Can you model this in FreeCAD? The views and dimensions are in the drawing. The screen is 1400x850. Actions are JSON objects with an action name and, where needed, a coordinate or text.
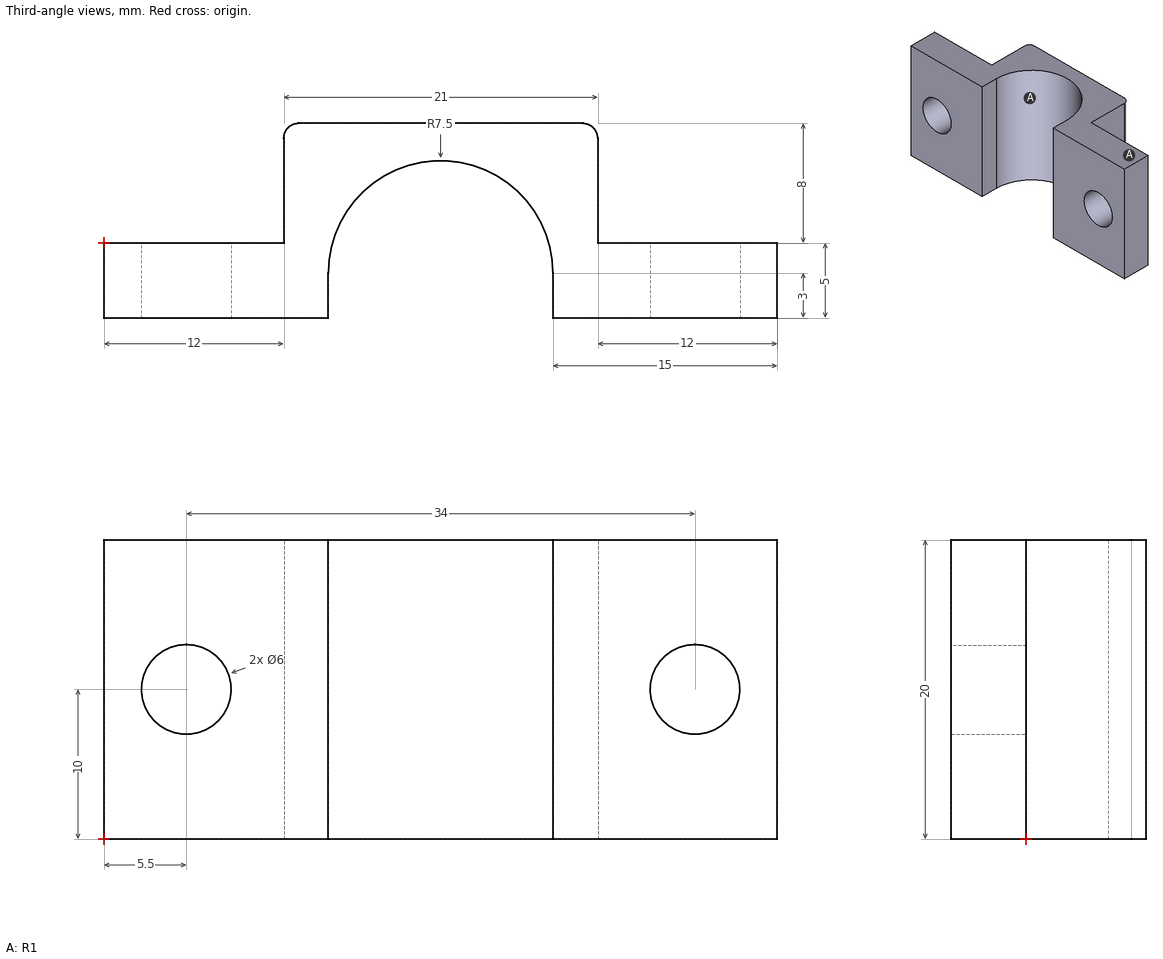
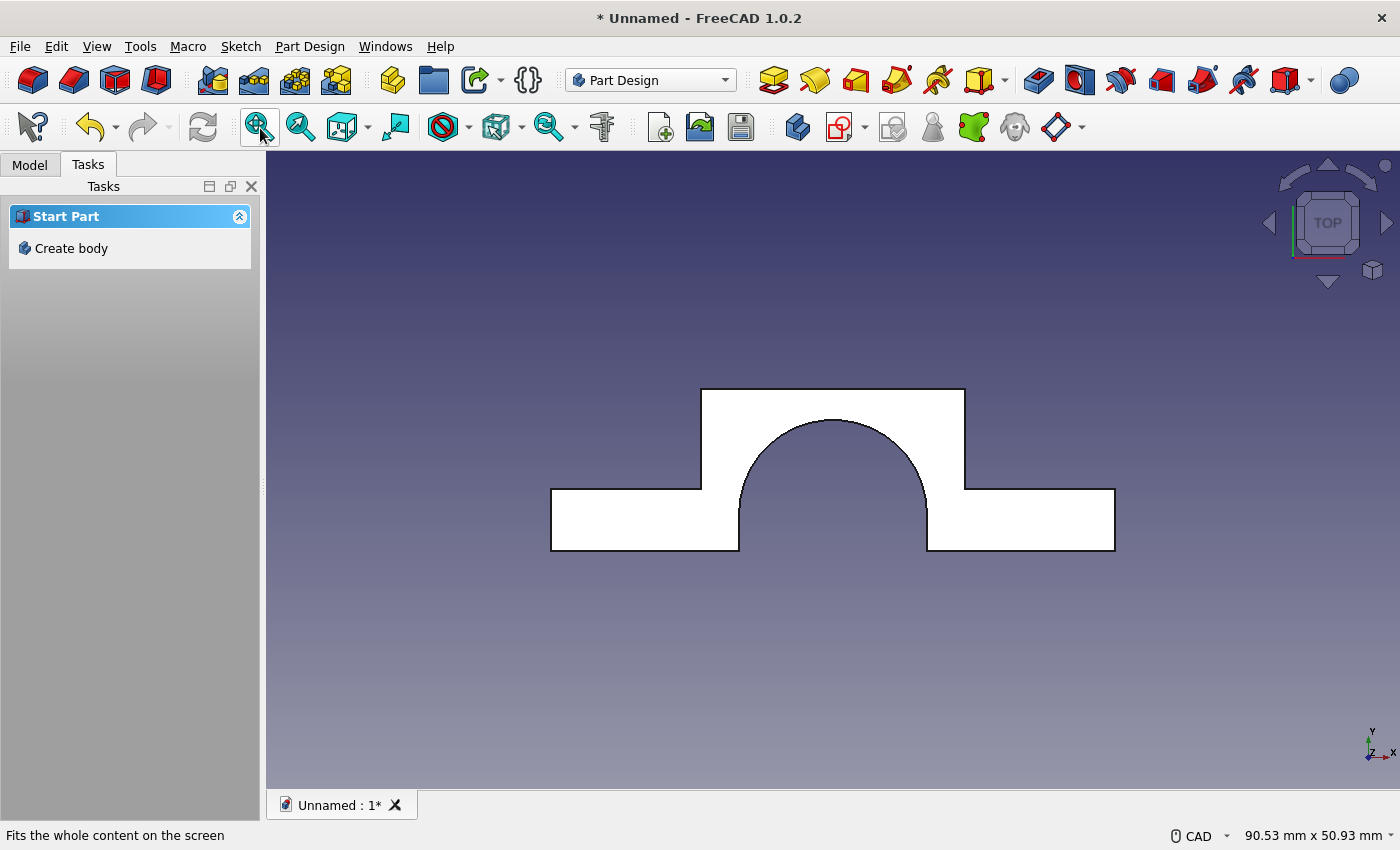
{"action": "key", "text": "1"}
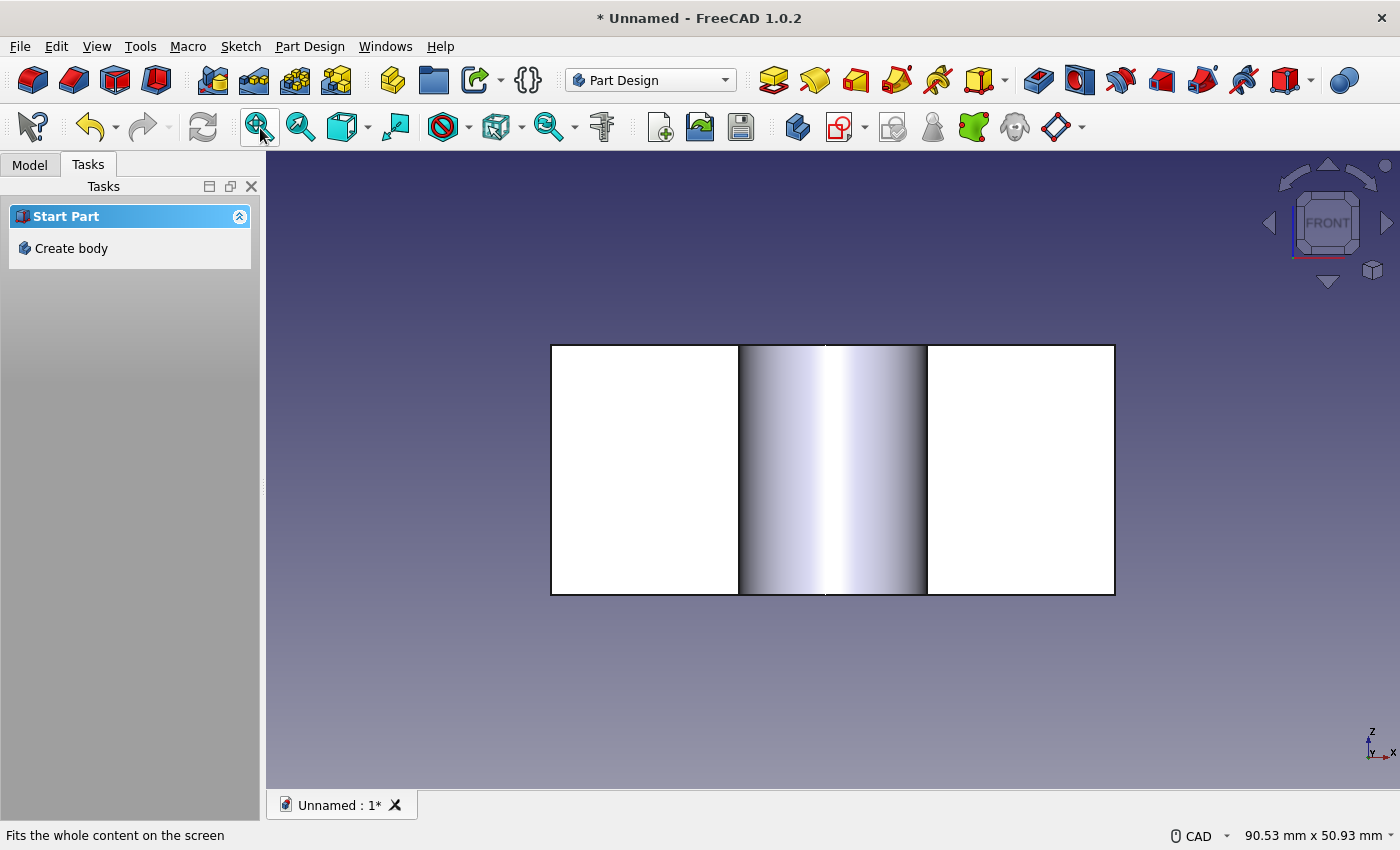
{"action": "key", "text": "3"}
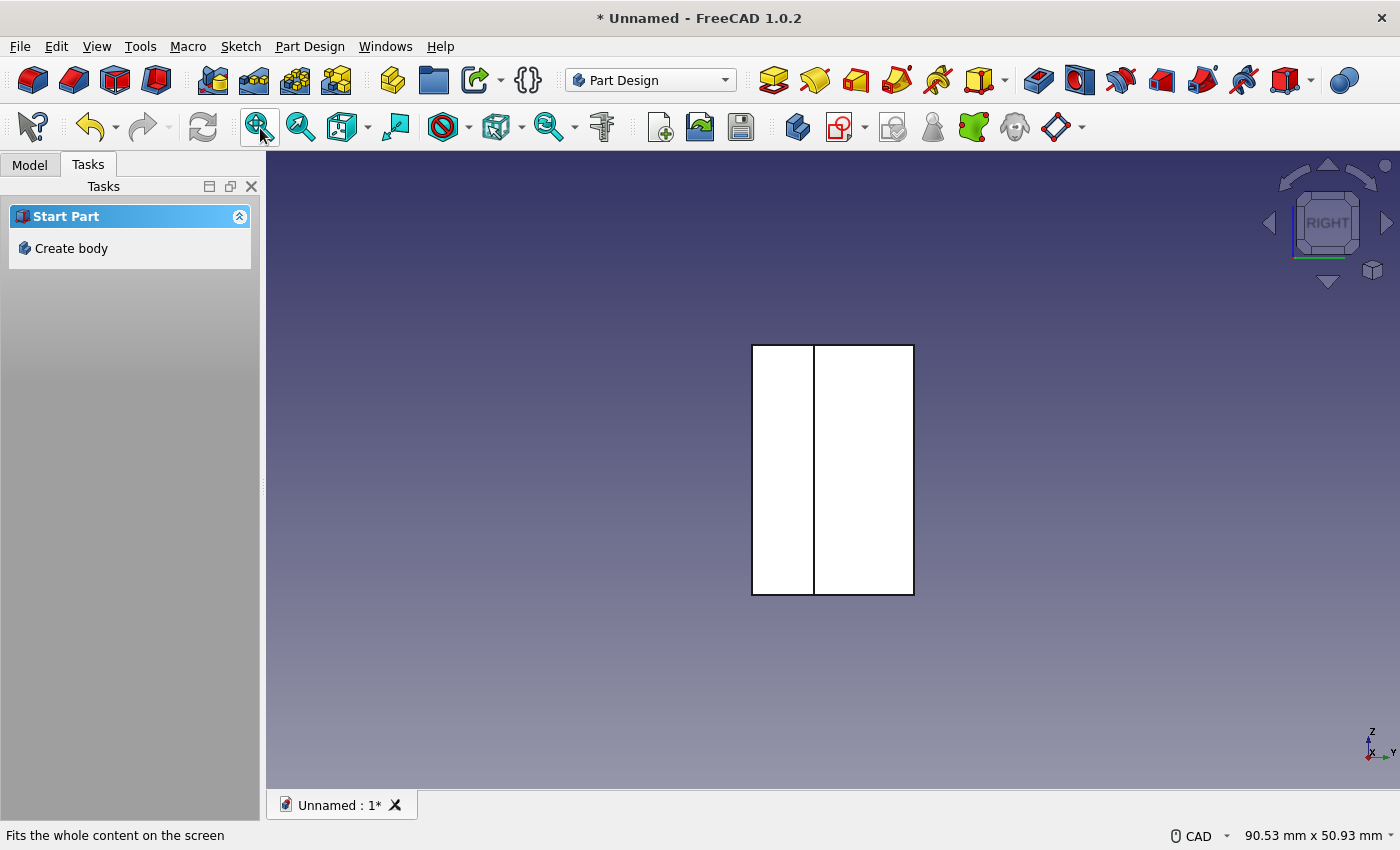
{"action": "left_click", "coordinate": [260, 128]}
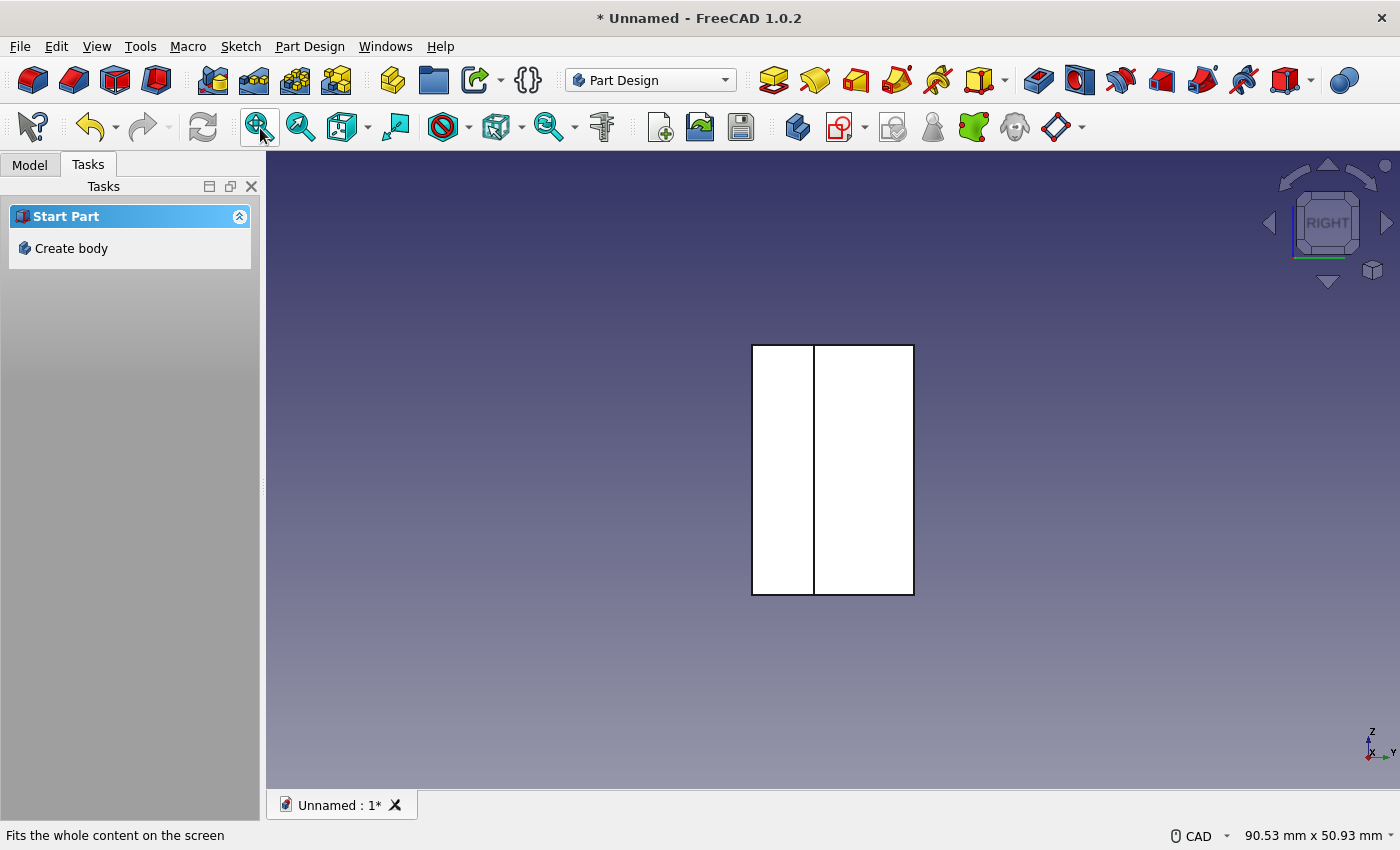
{"action": "left_click", "coordinate": [914, 469]}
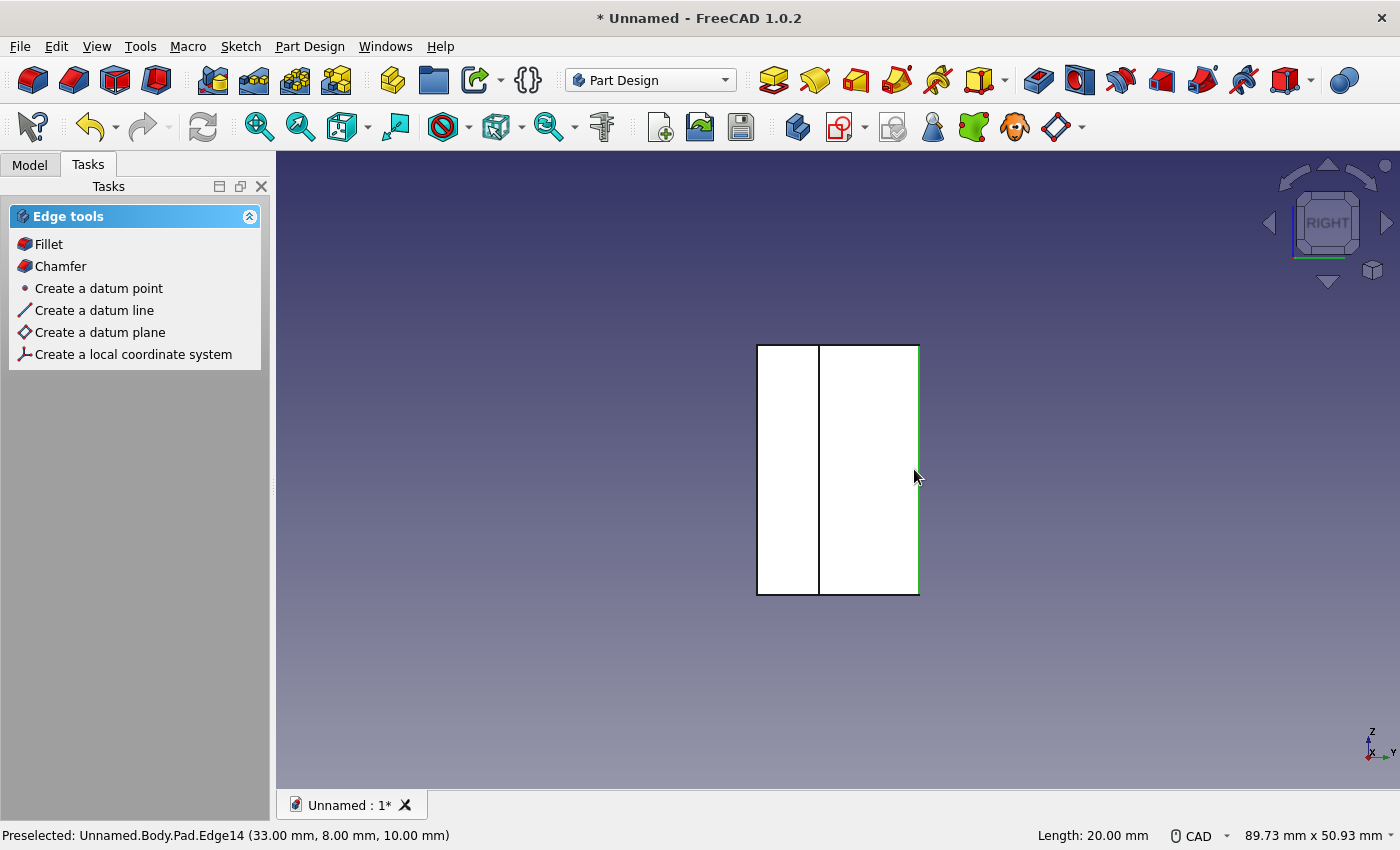
{"action": "key", "text": "5"}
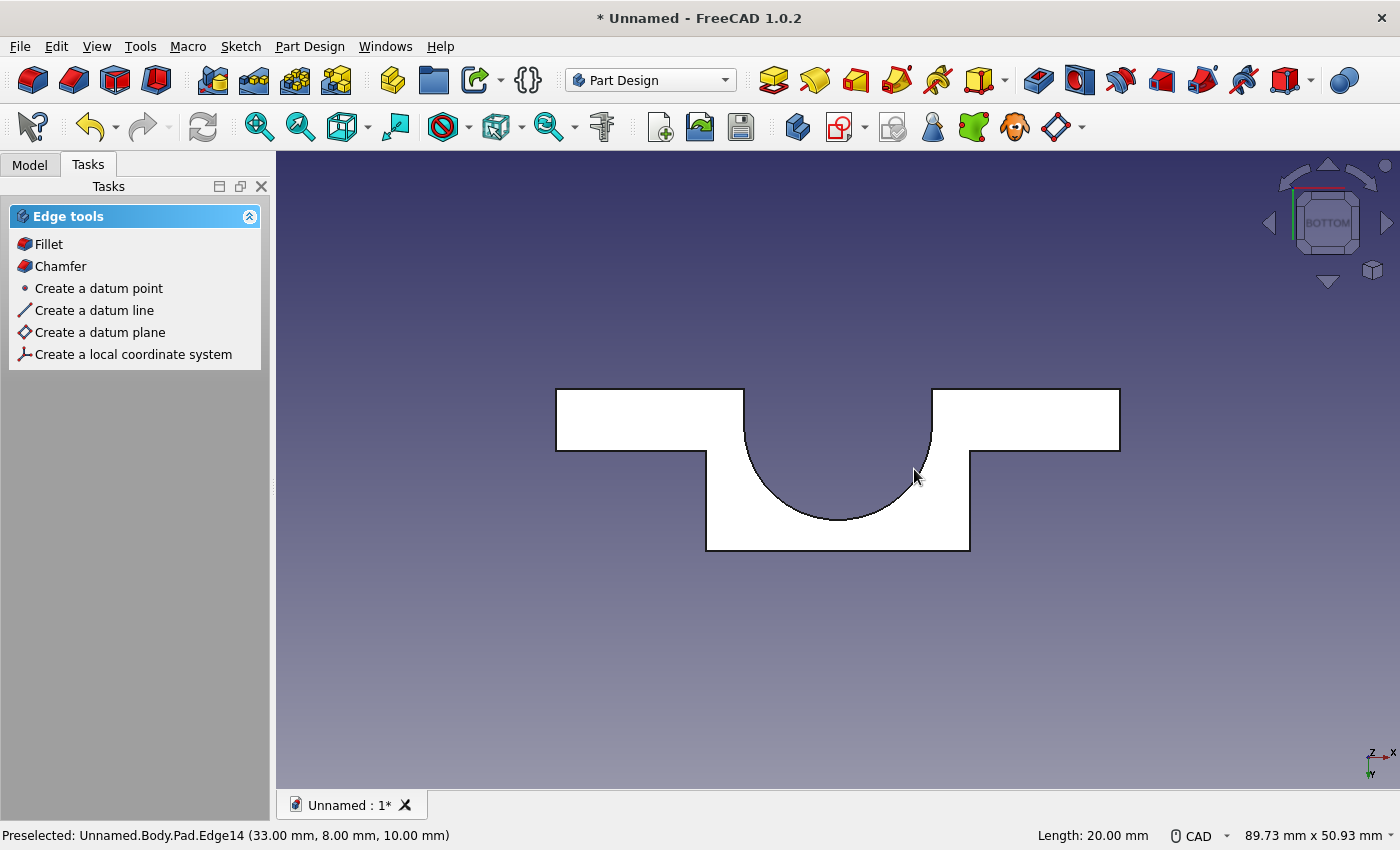
{"action": "key", "text": "4"}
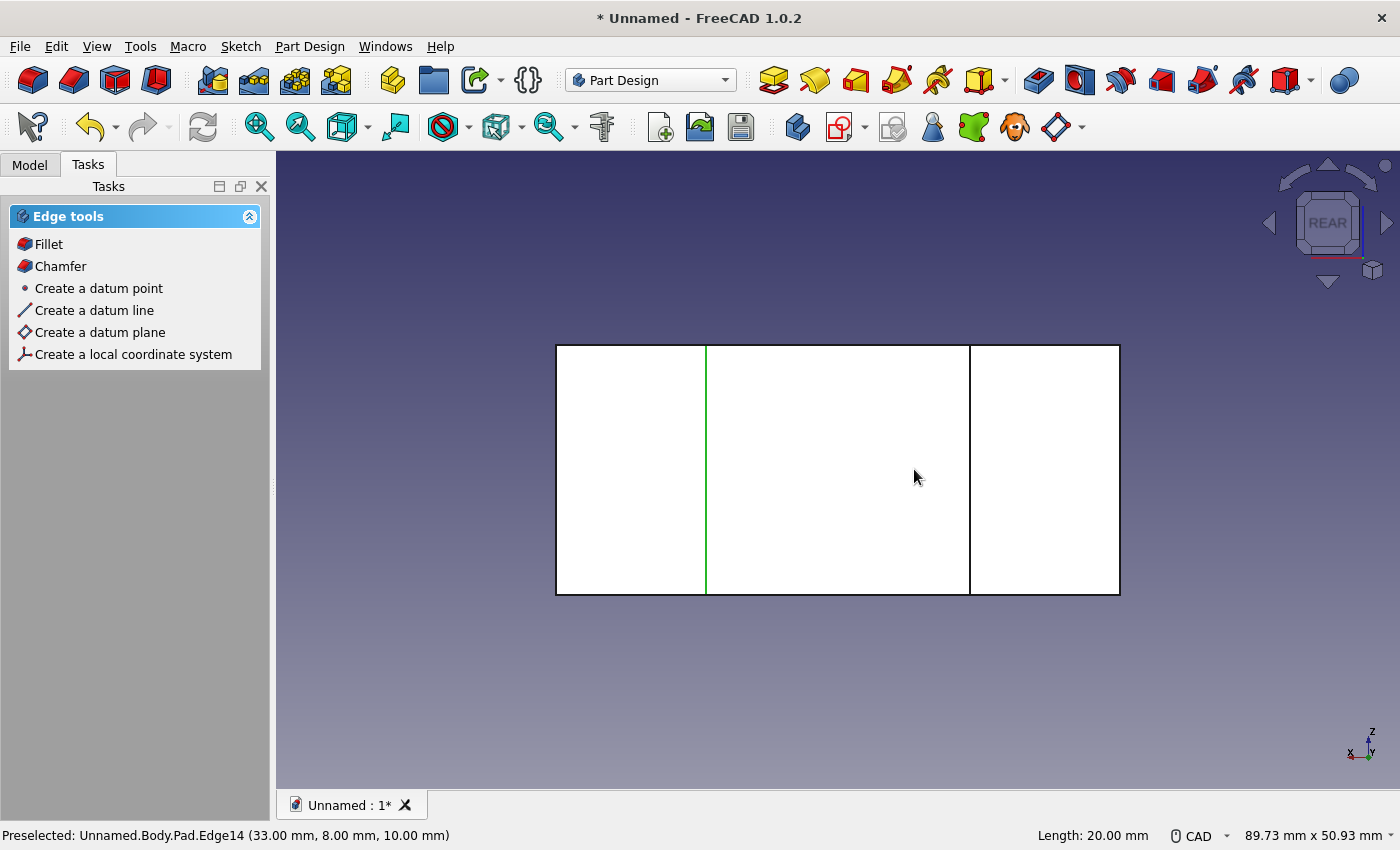
{"action": "left_click", "coordinate": [970, 469], "text": "ctrl"}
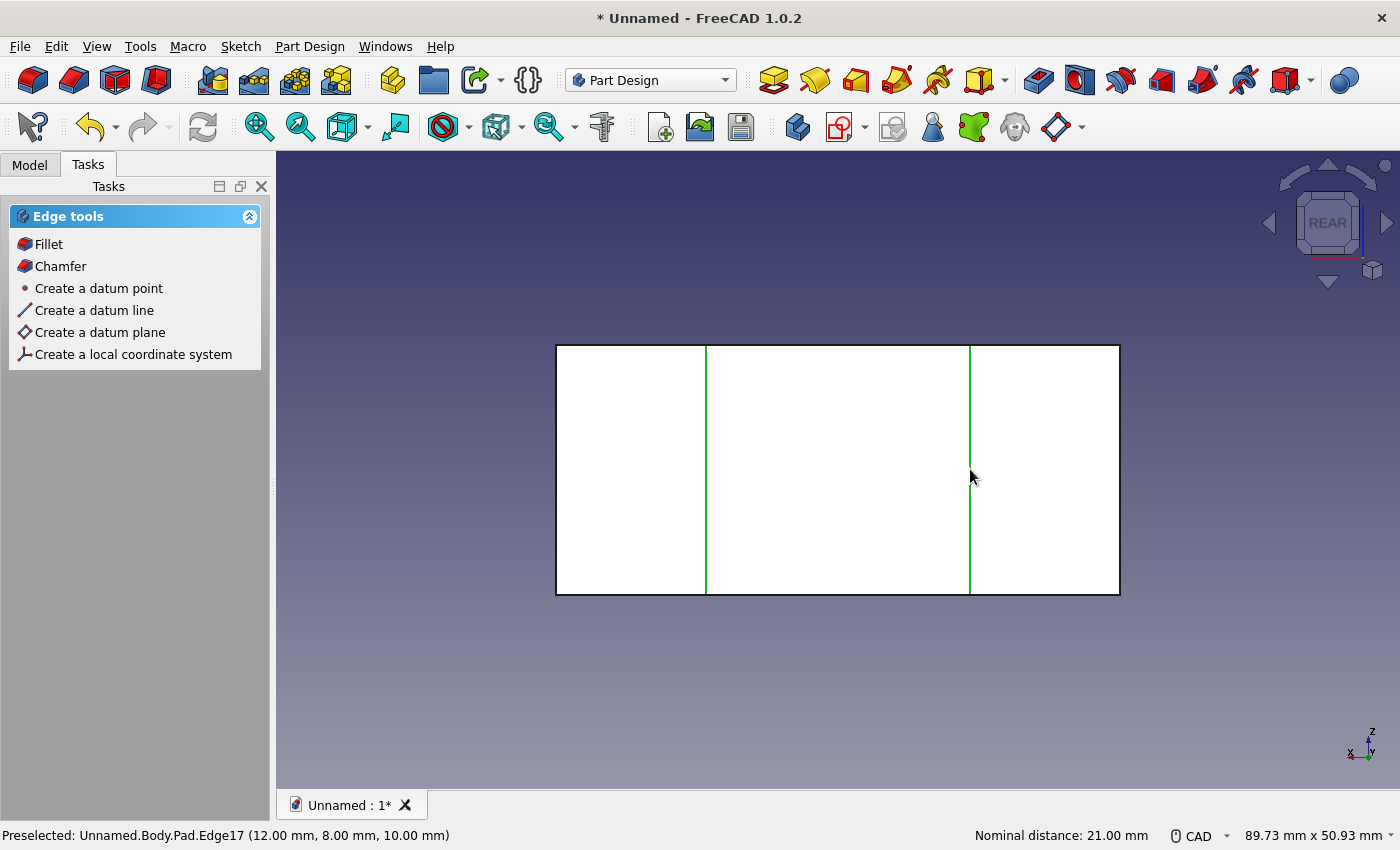
{"action": "left_click", "coordinate": [33, 80]}